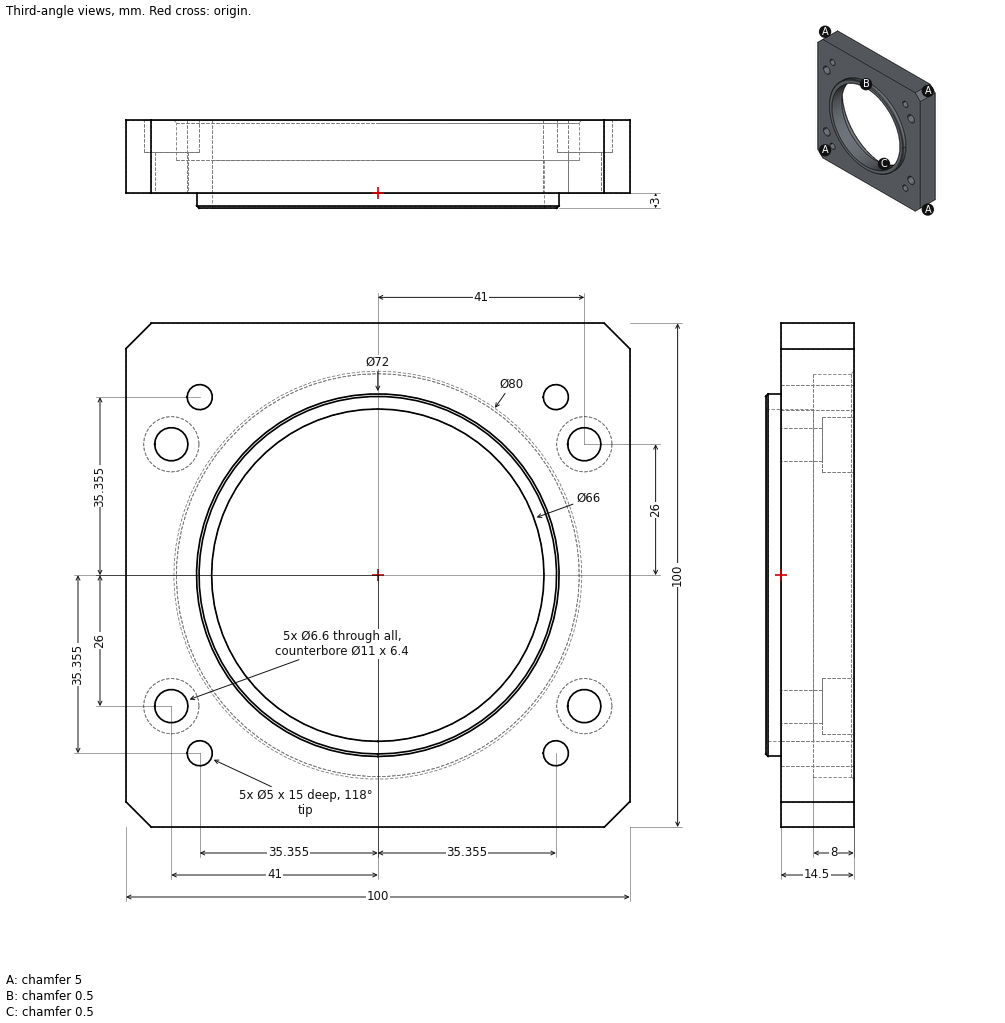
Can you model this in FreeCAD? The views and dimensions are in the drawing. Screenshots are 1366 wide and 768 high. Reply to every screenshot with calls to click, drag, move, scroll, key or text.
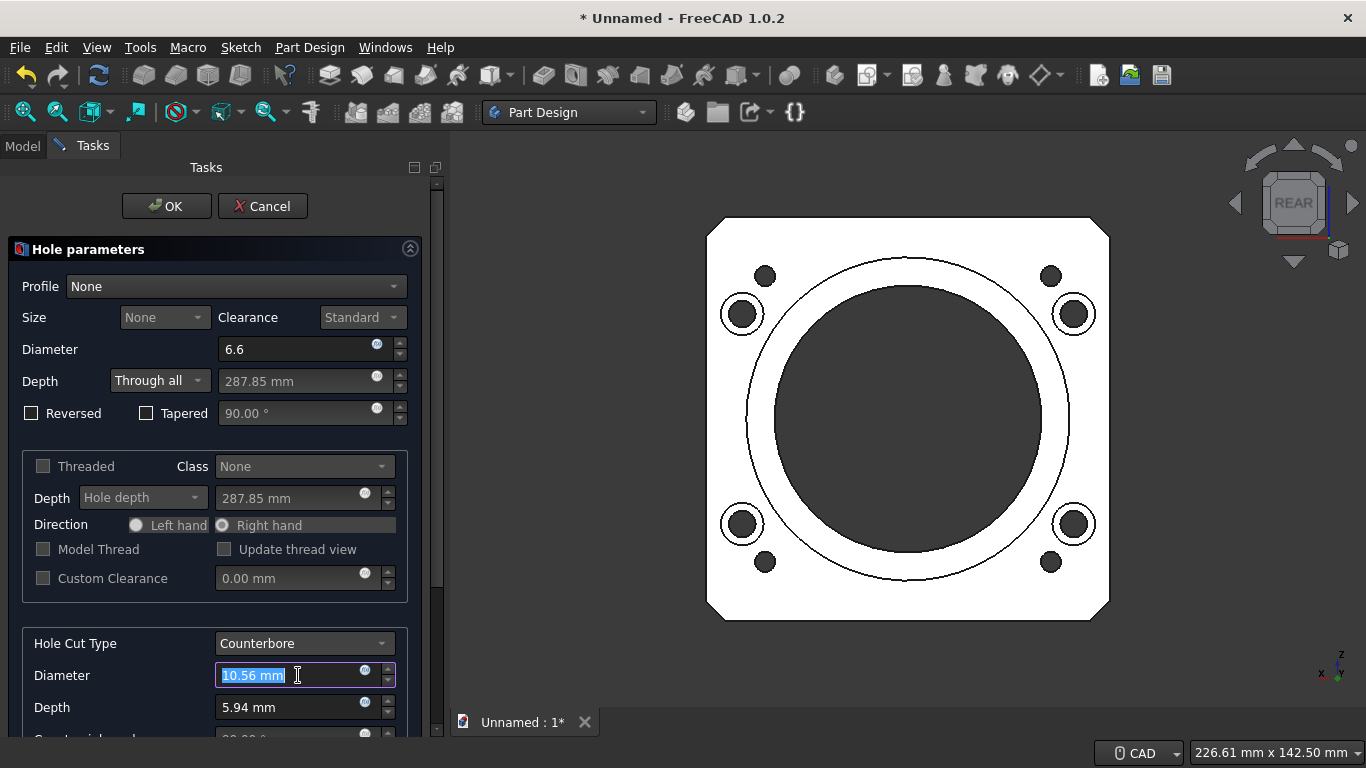
text(11)
key(Tab)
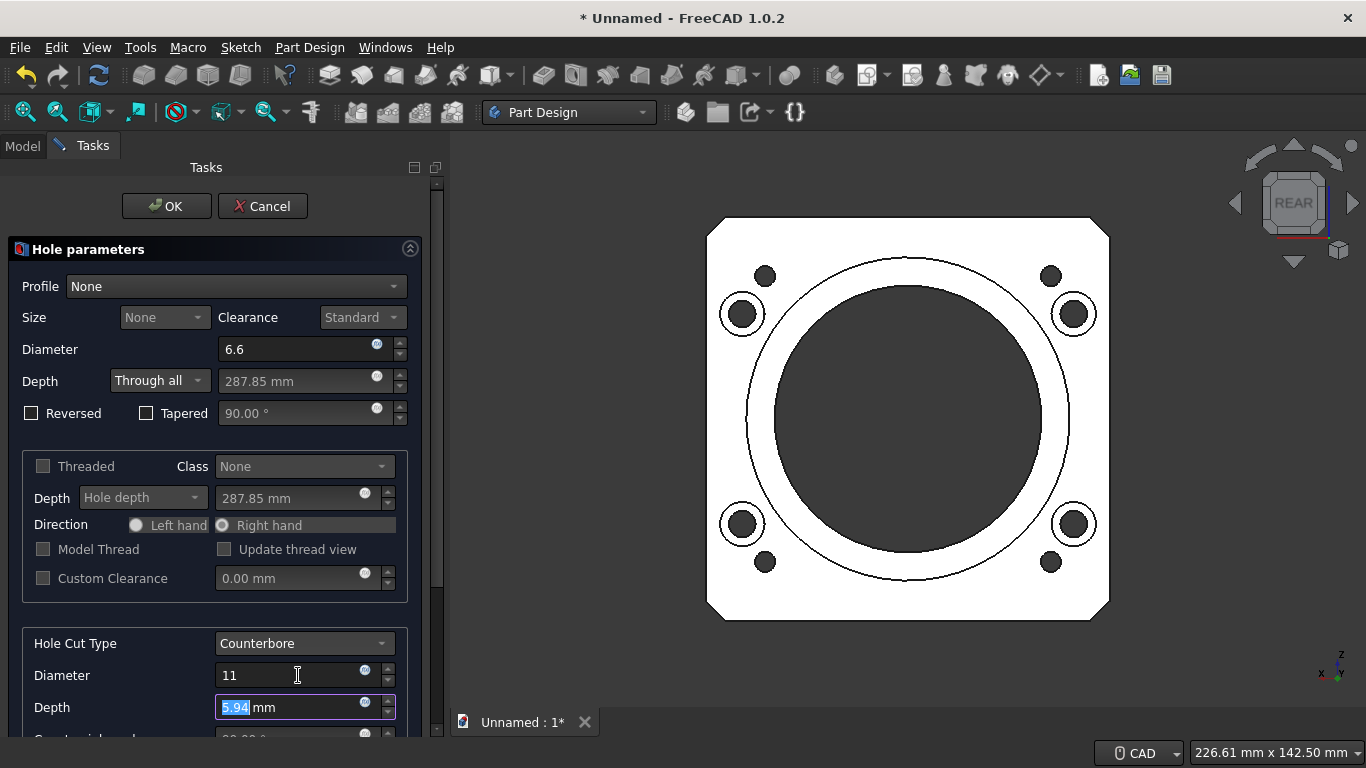
text(6.4)
key(Tab)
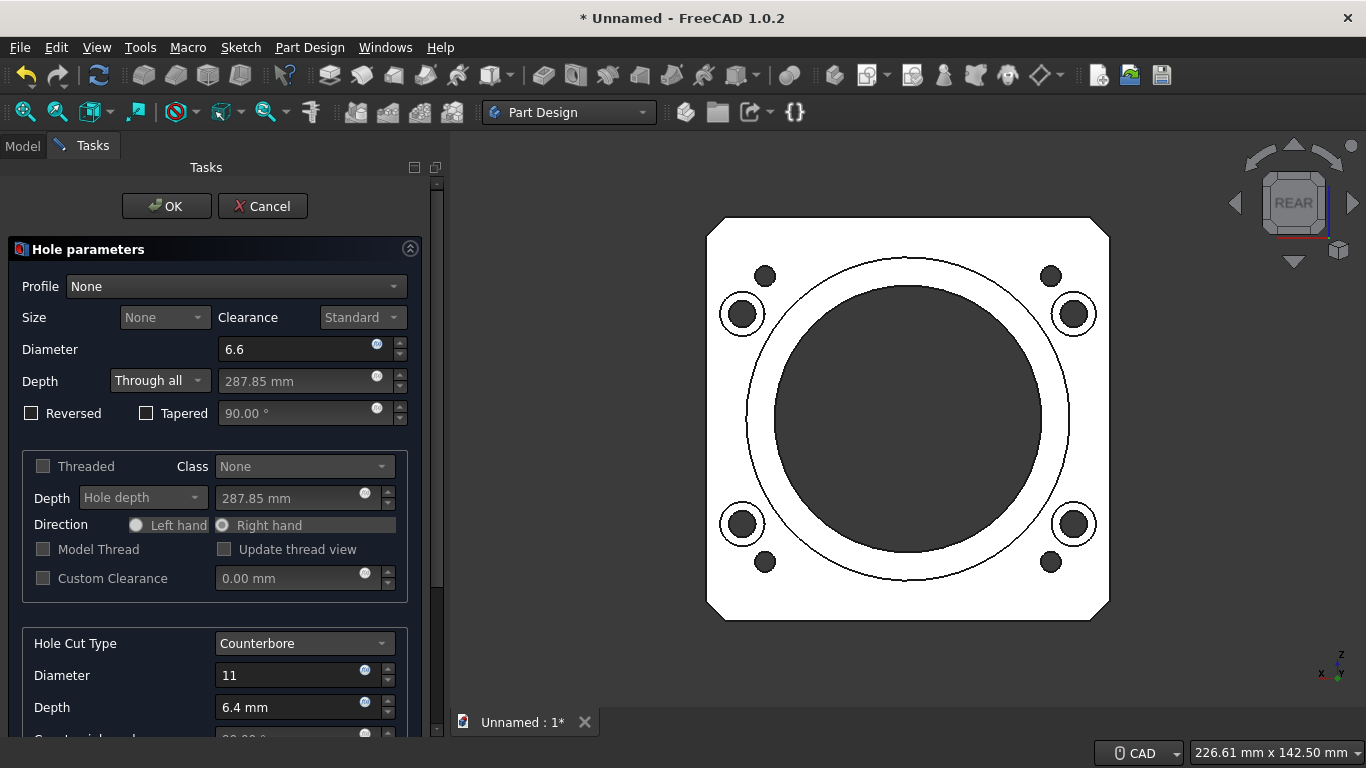
click(167, 206)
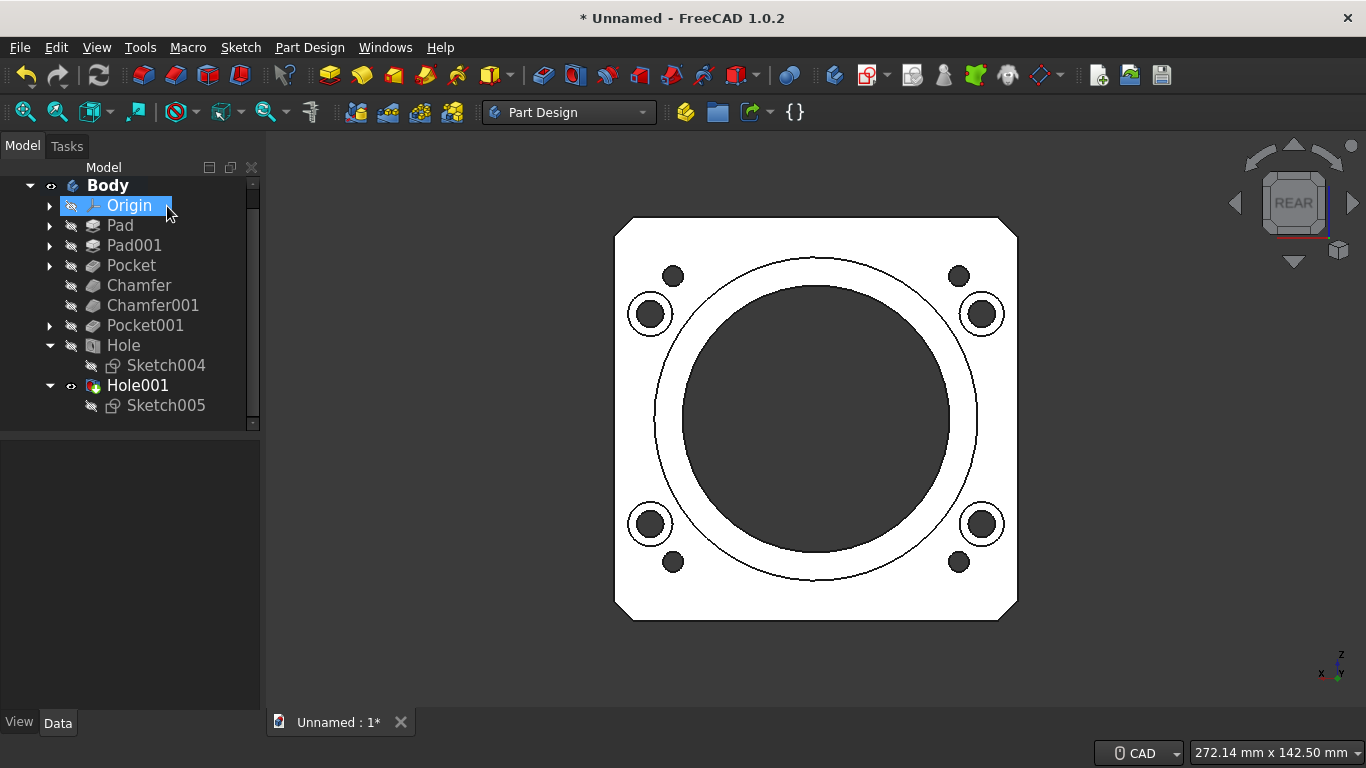
click(947, 323)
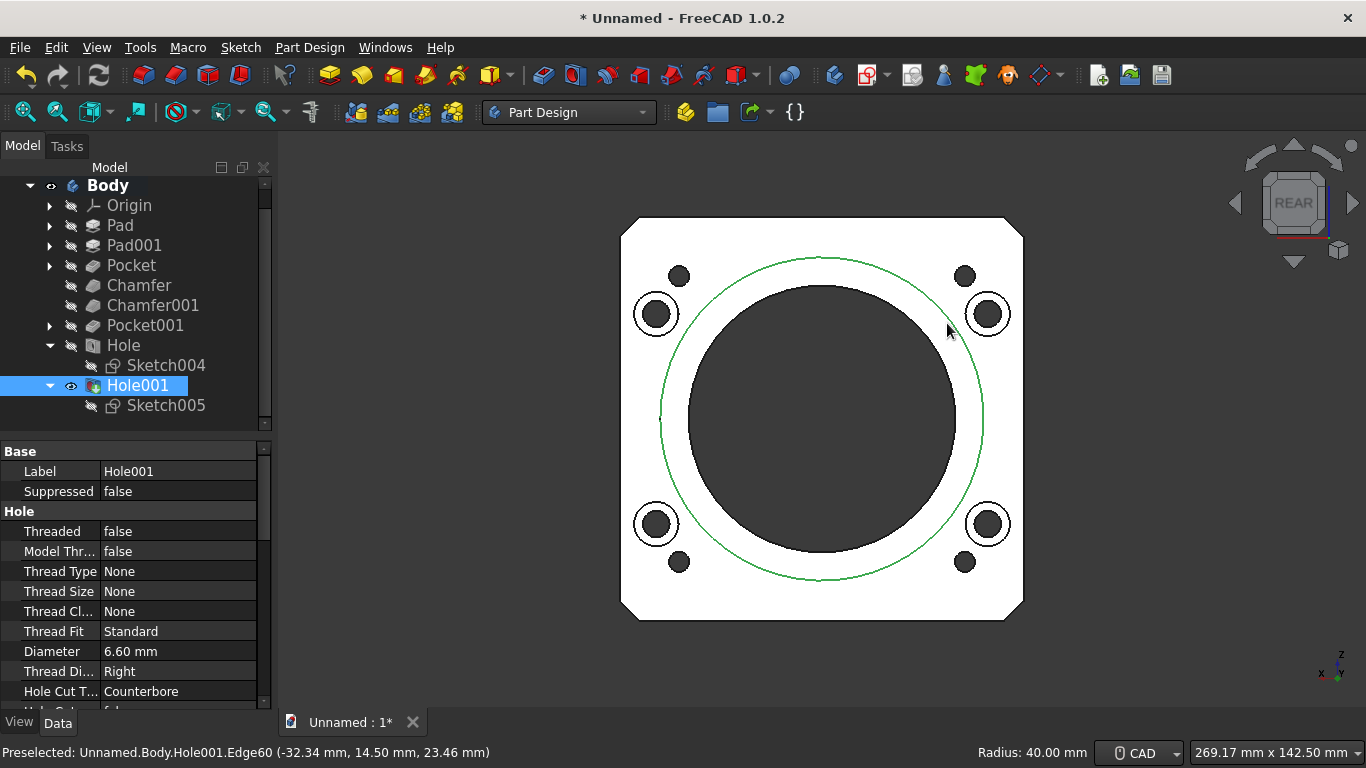
click(176, 76)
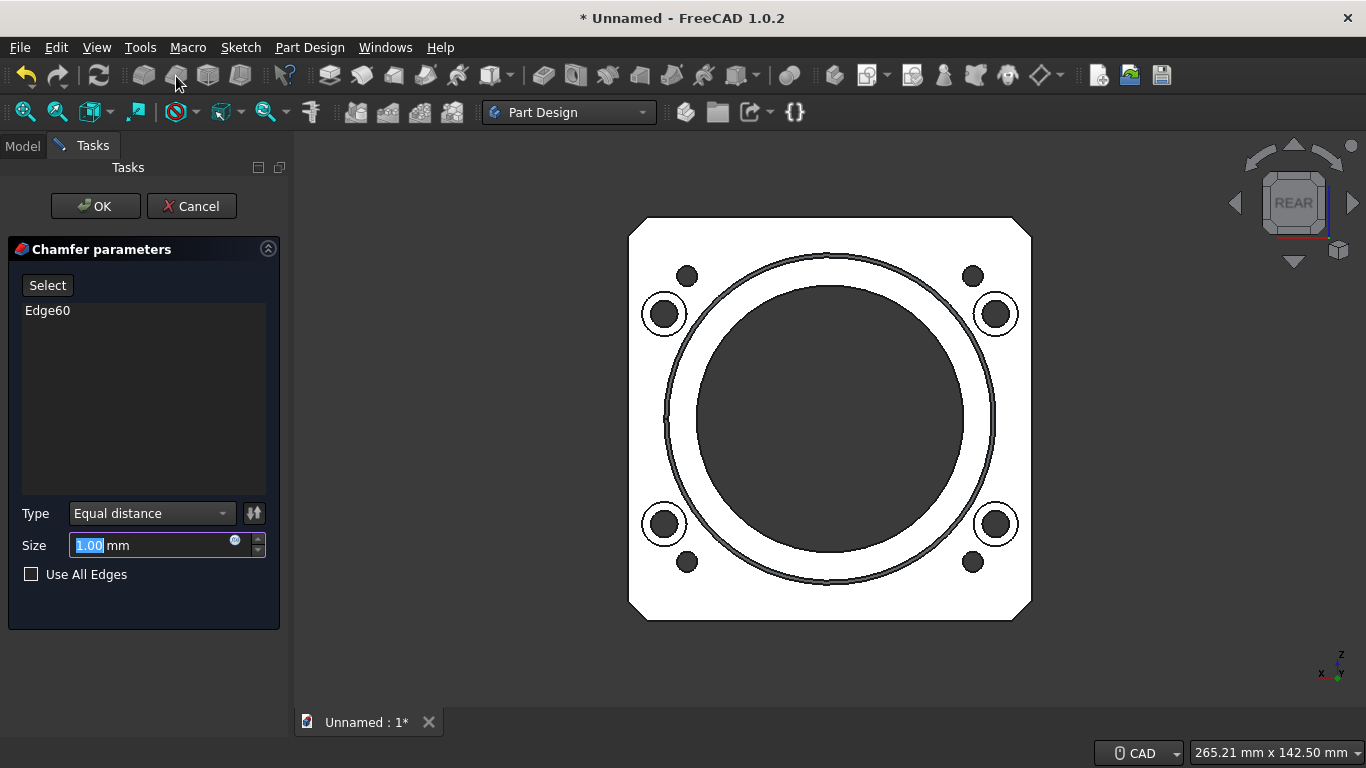
text(0.5)
key(Tab)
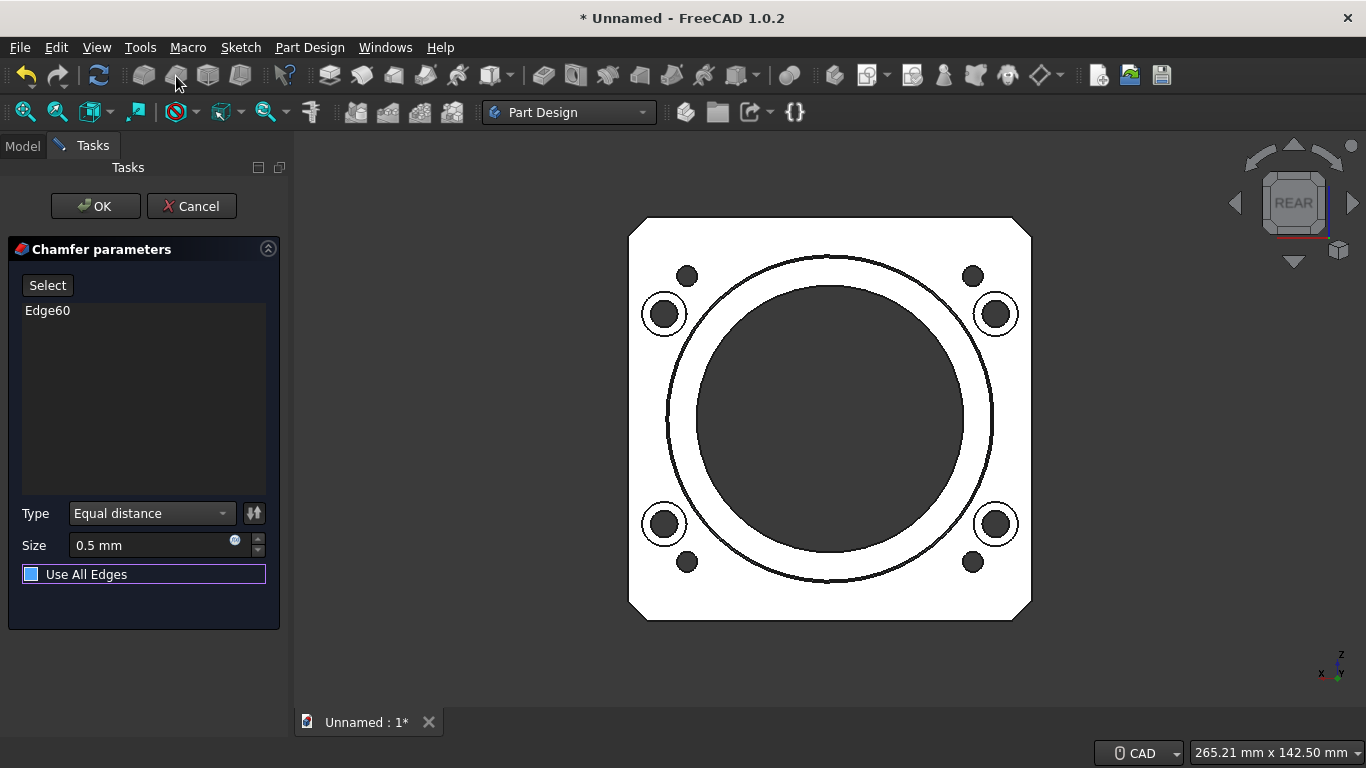
click(96, 206)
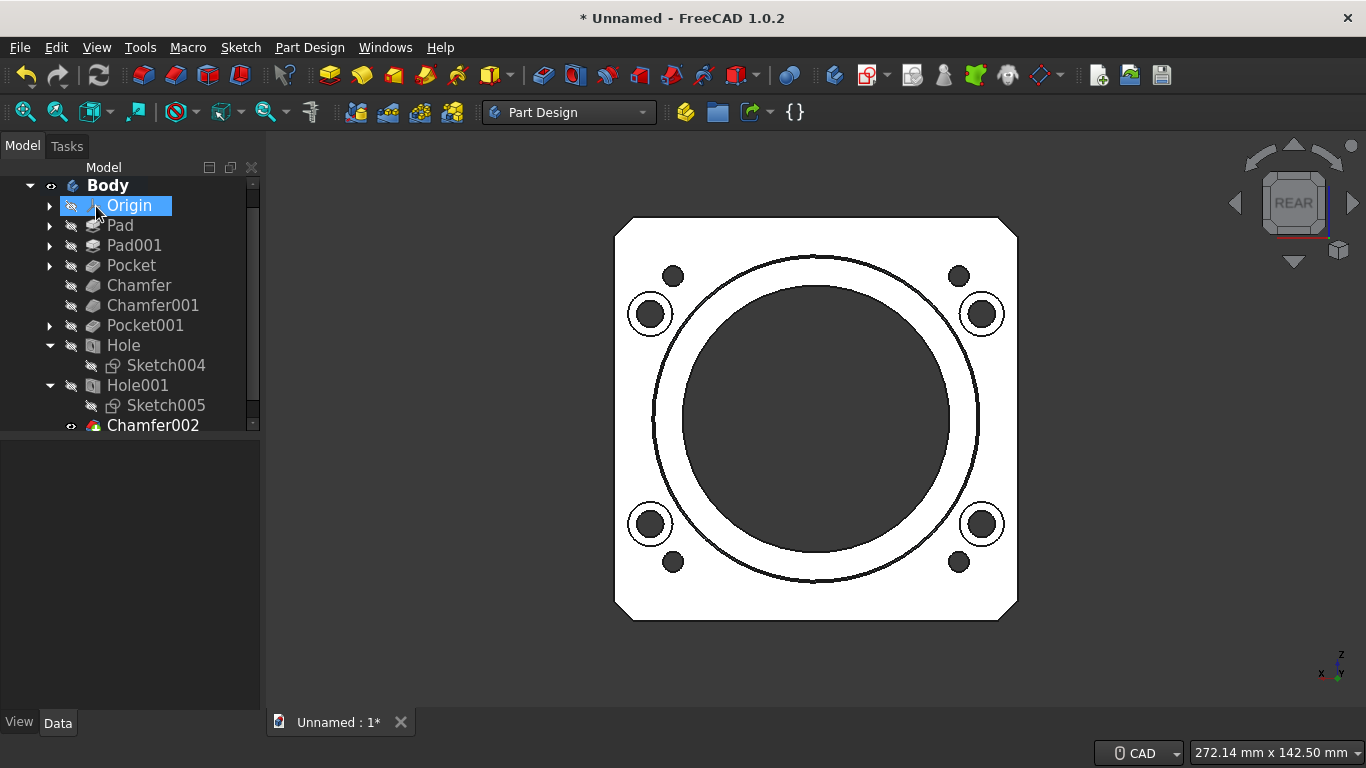
key(0)